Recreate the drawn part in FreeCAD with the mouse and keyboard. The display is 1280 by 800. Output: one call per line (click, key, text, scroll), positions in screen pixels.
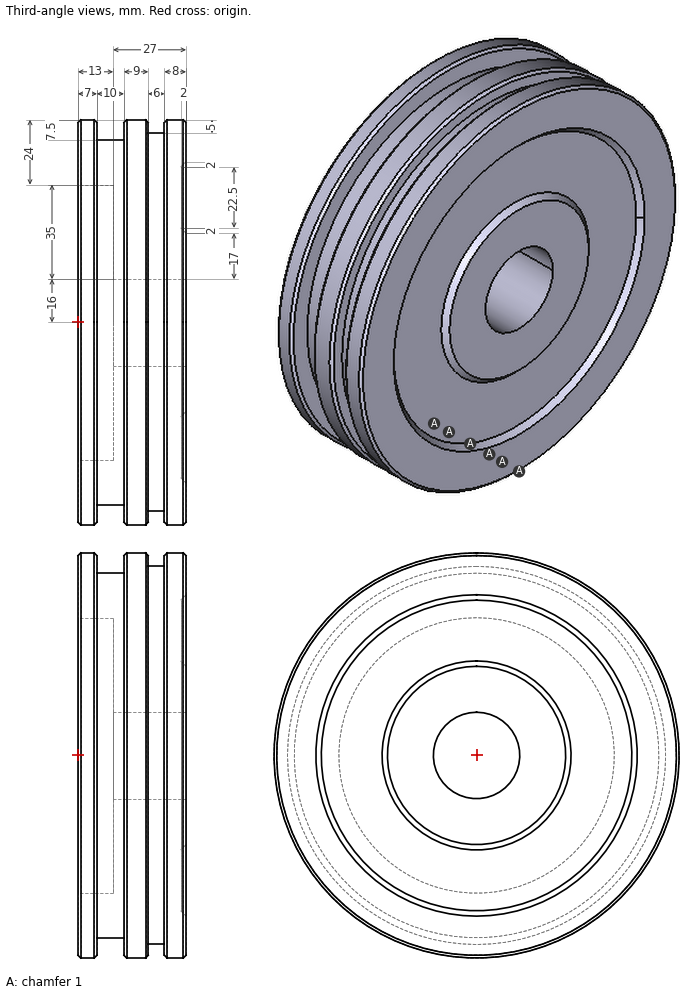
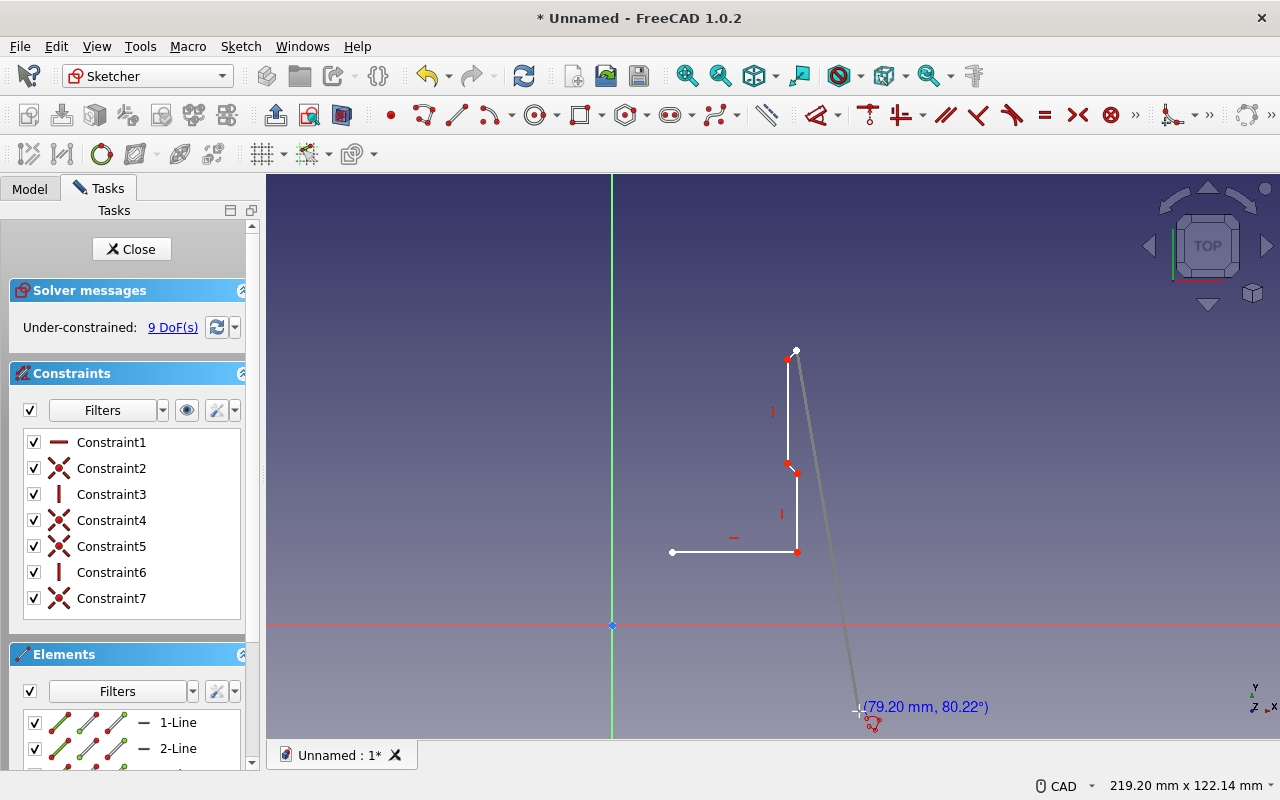
click(797, 278)
click(760, 278)
click(760, 301)
click(732, 301)
click(732, 278)
click(691, 278)
click(691, 313)
click(645, 313)
click(645, 278)
click(612, 278)
click(621, 389)
click(672, 389)
click(672, 552)
key(Escape)
key(Escape)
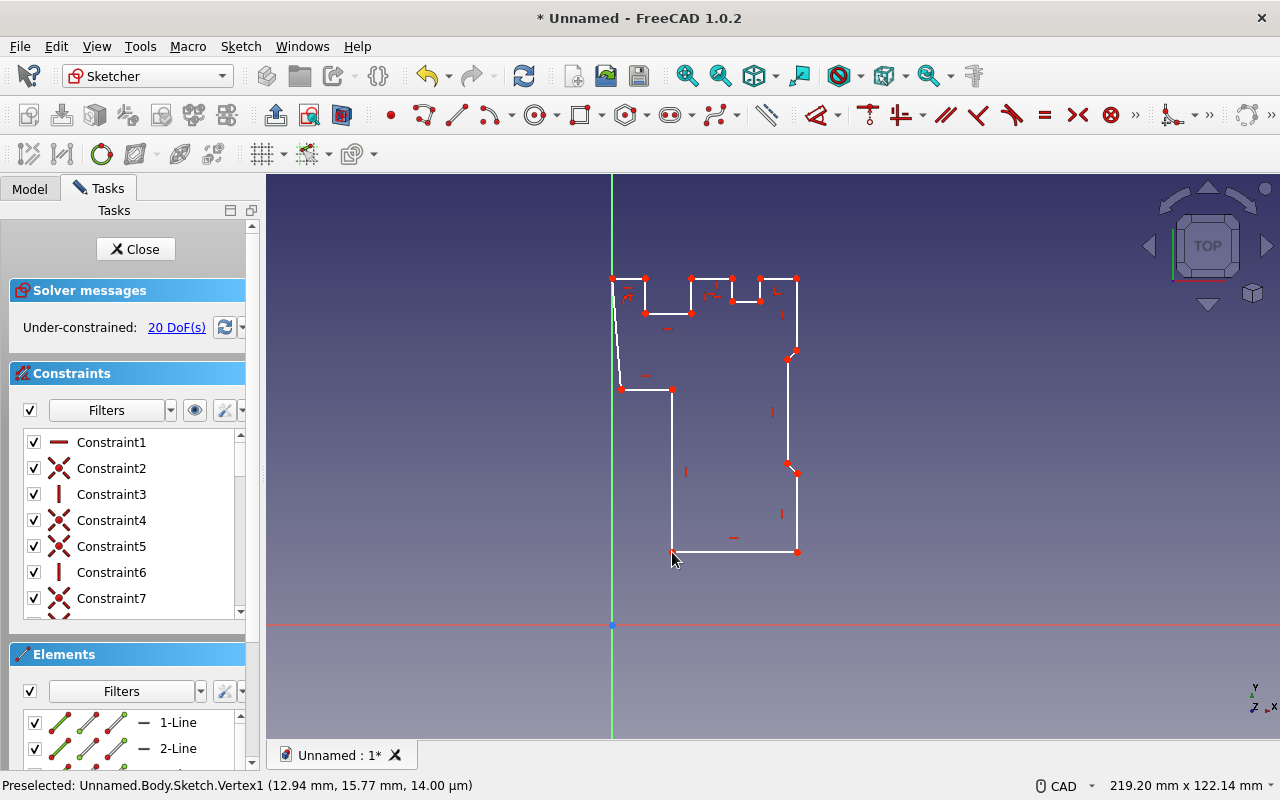
click(615, 312)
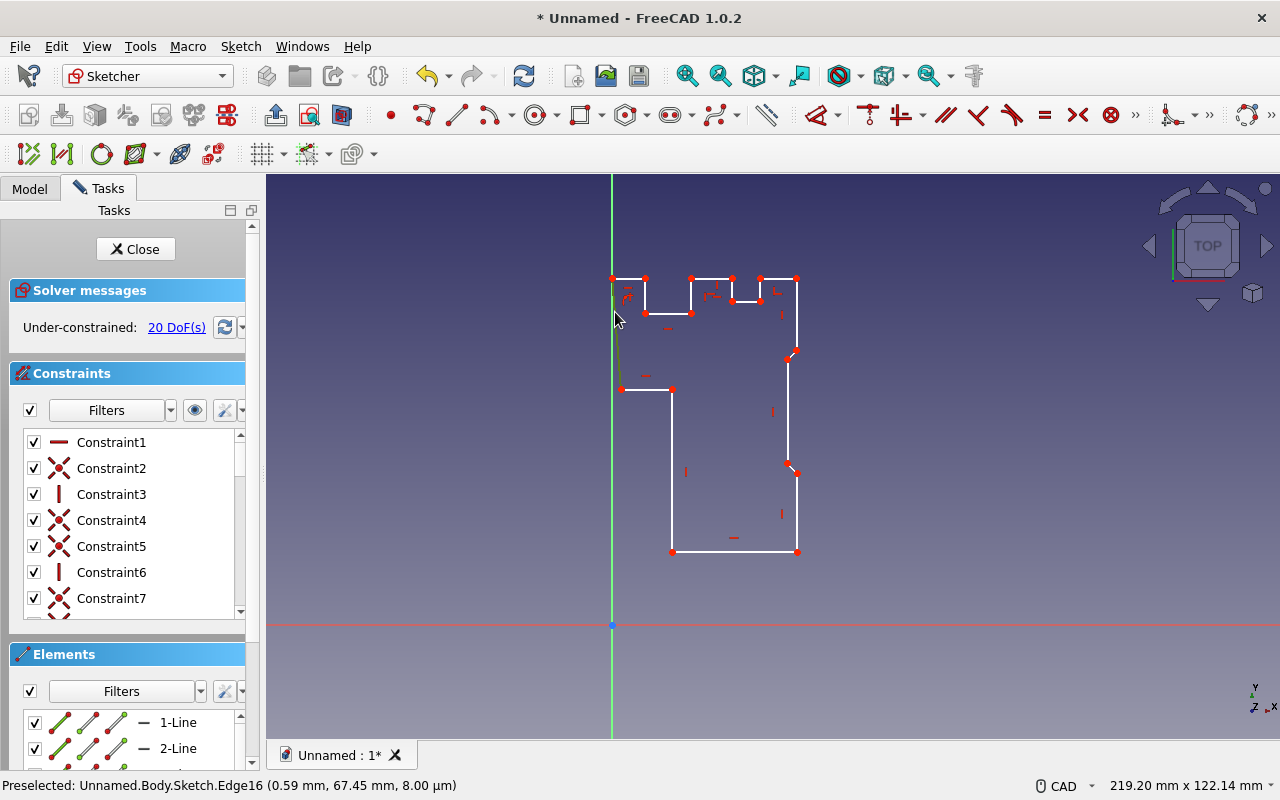
click(922, 116)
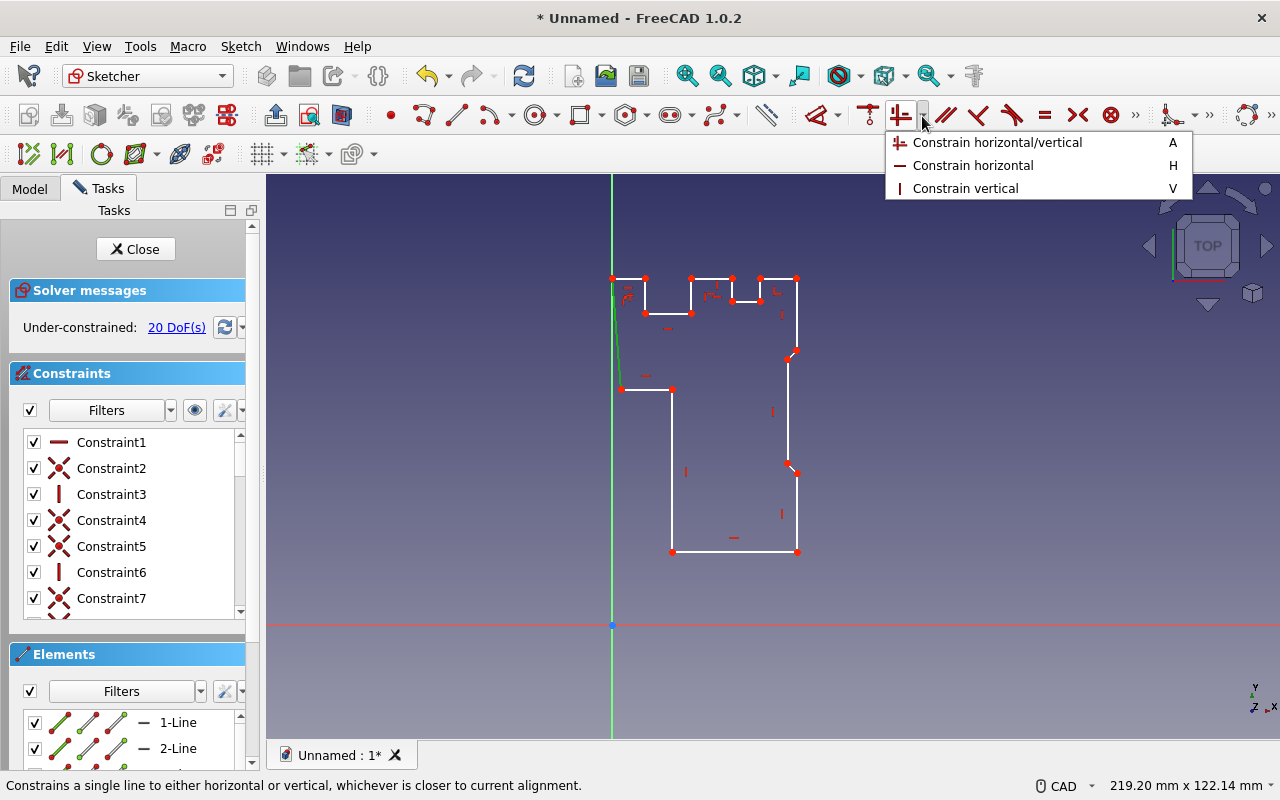
click(1039, 188)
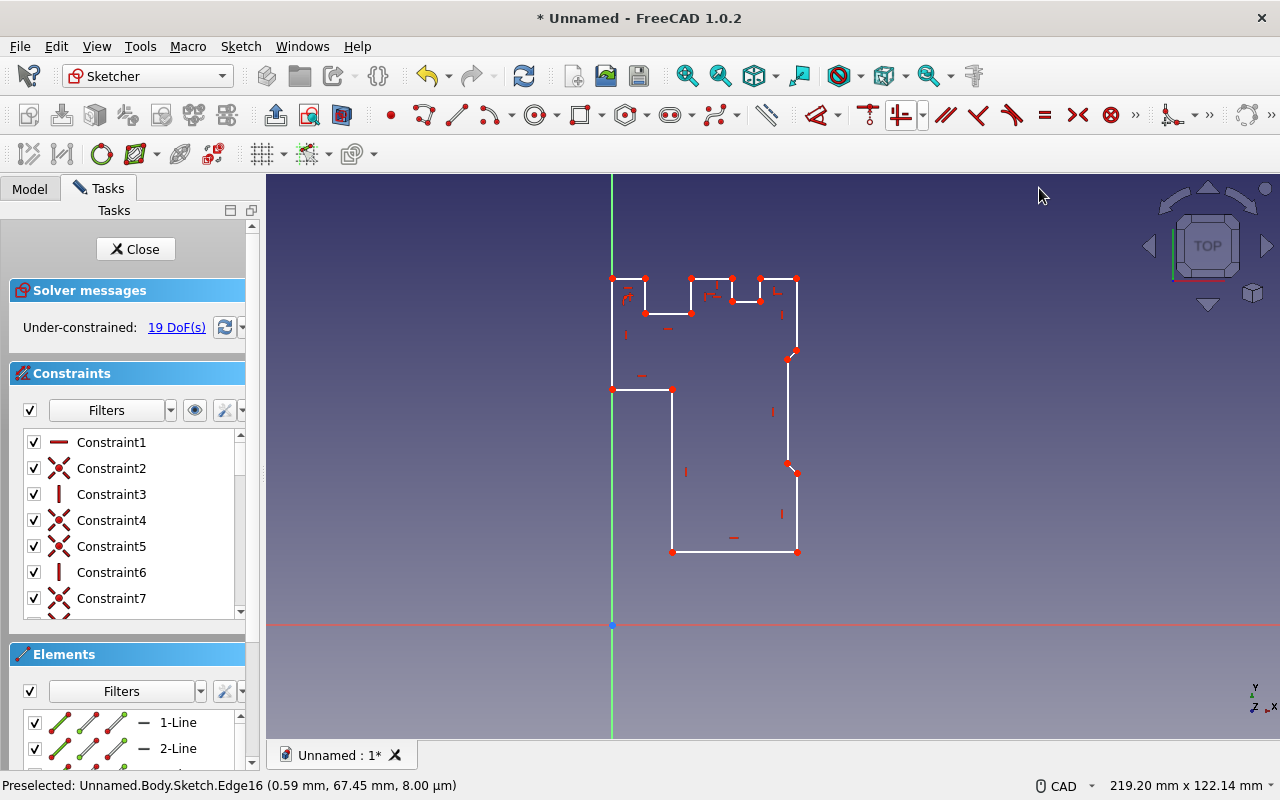
click(816, 116)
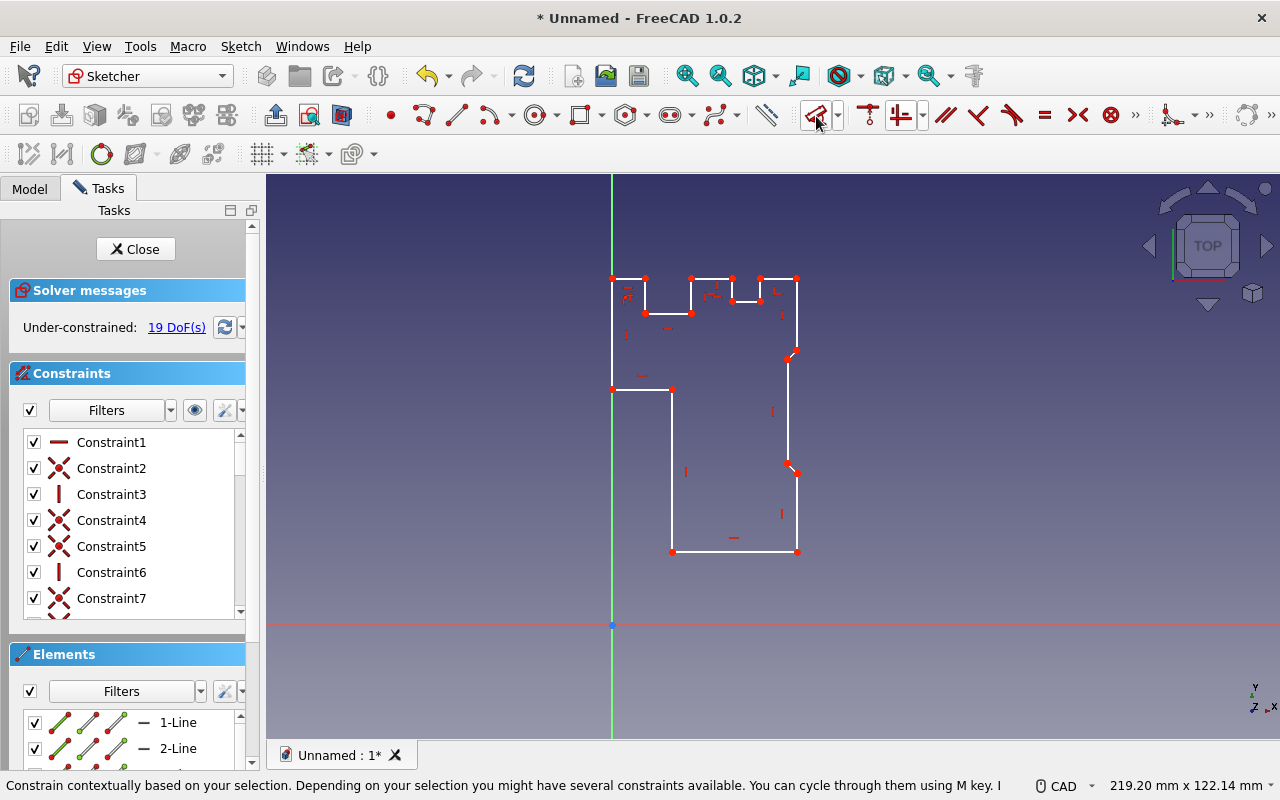
scroll(786, 279, up, 2)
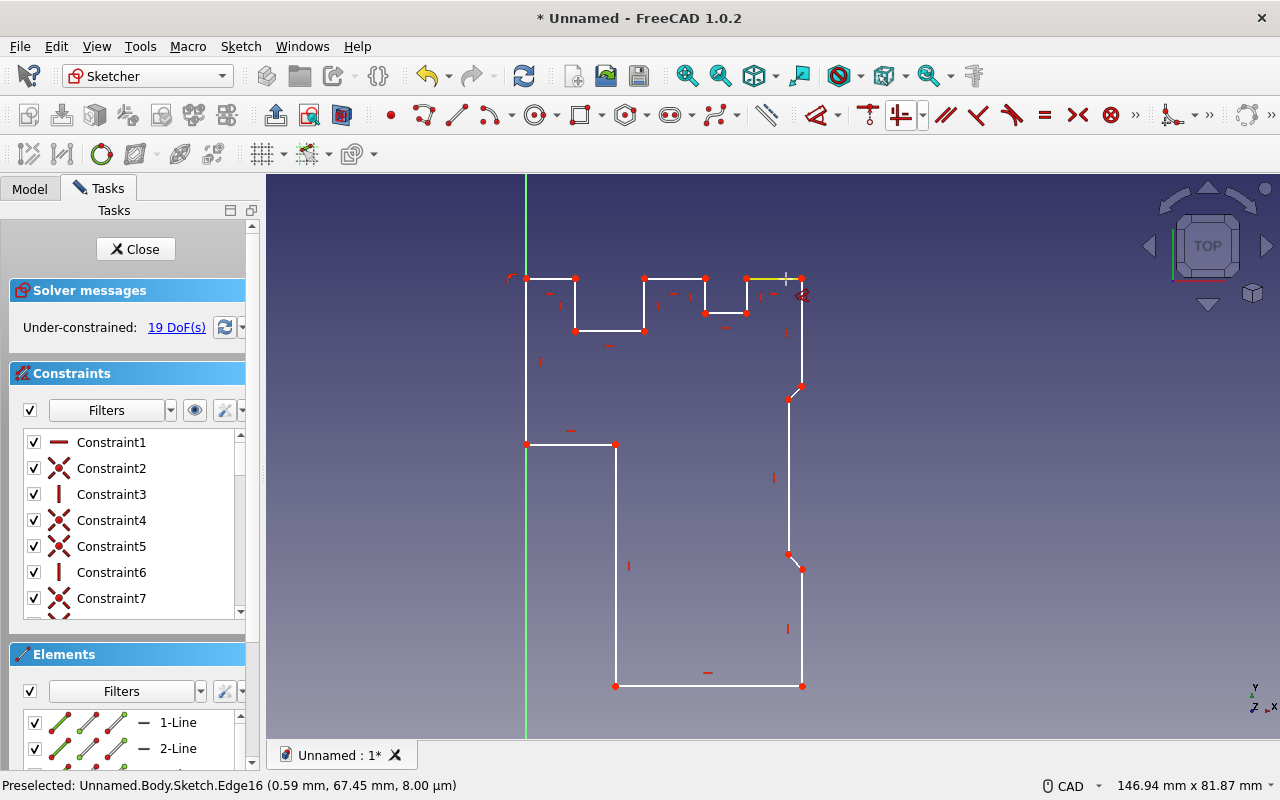
click(785, 279)
click(774, 245)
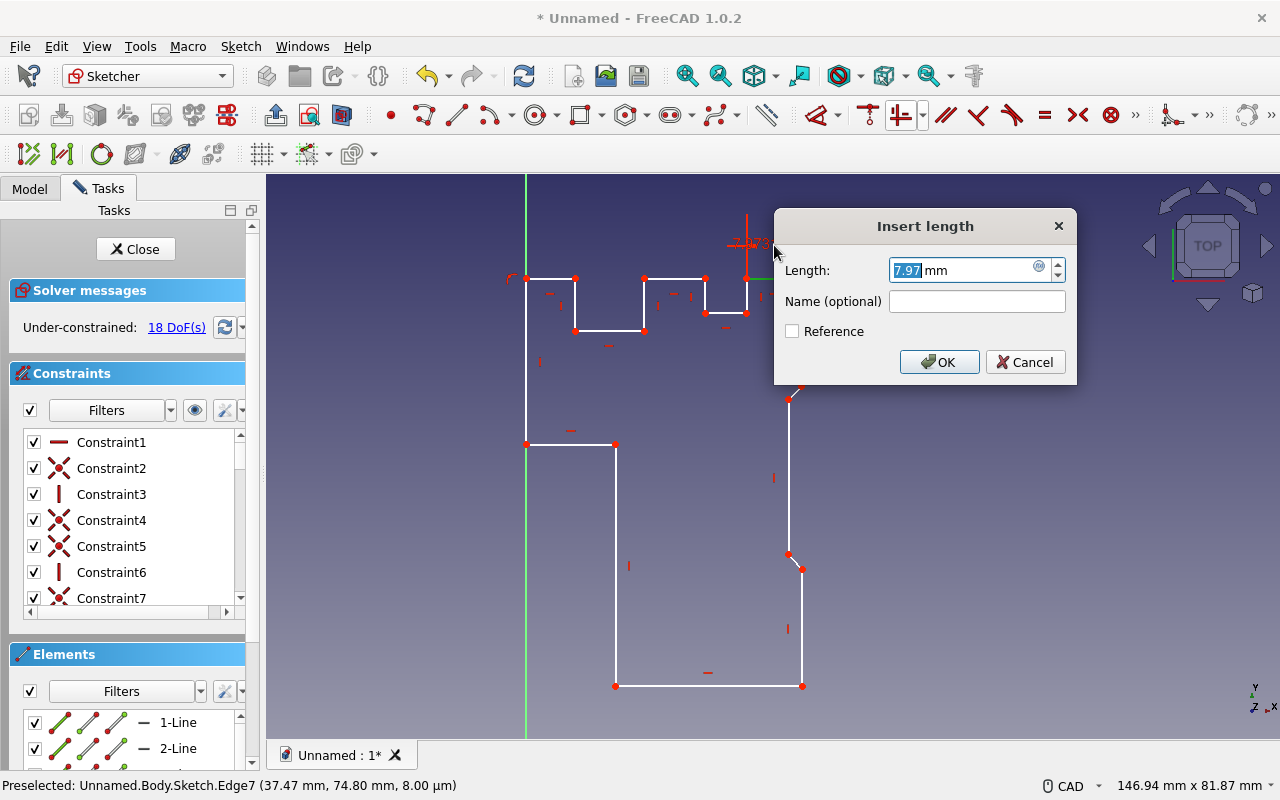
text(8)
key(Return)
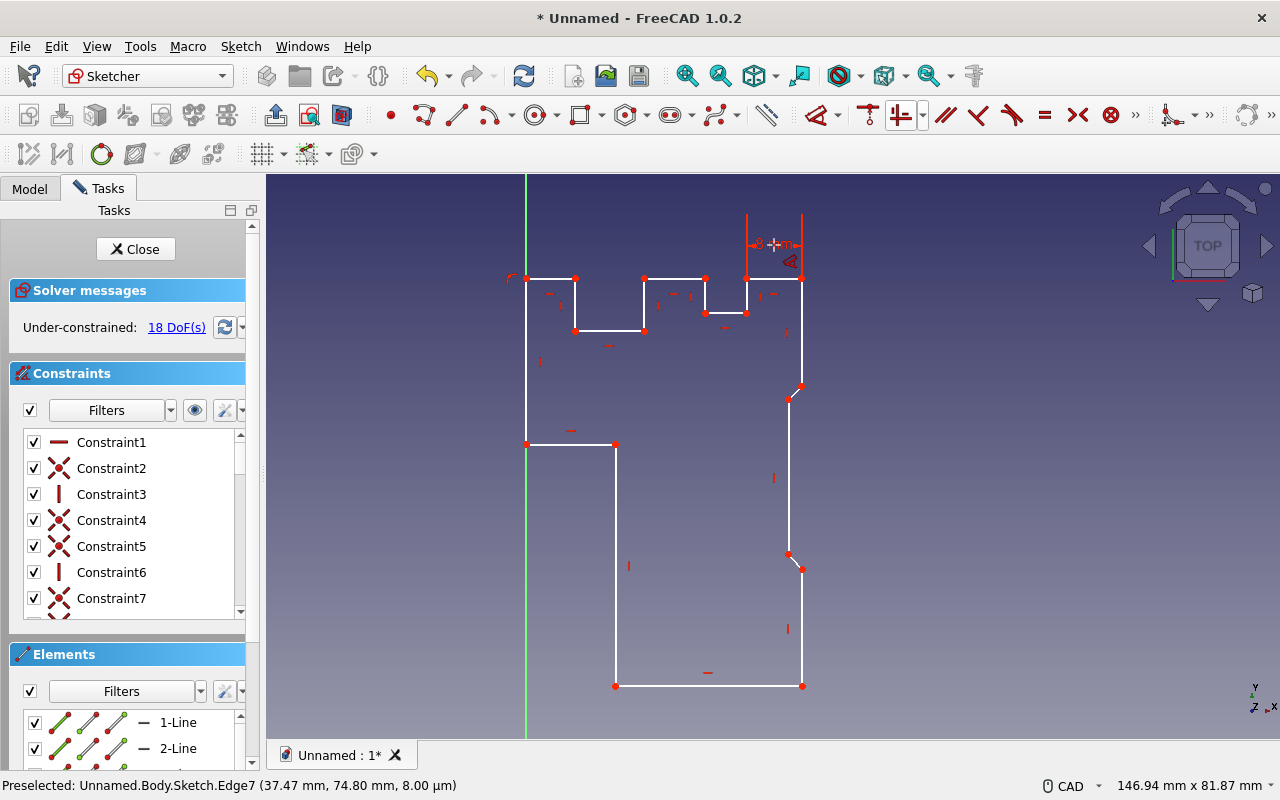
scroll(747, 289, up, 2)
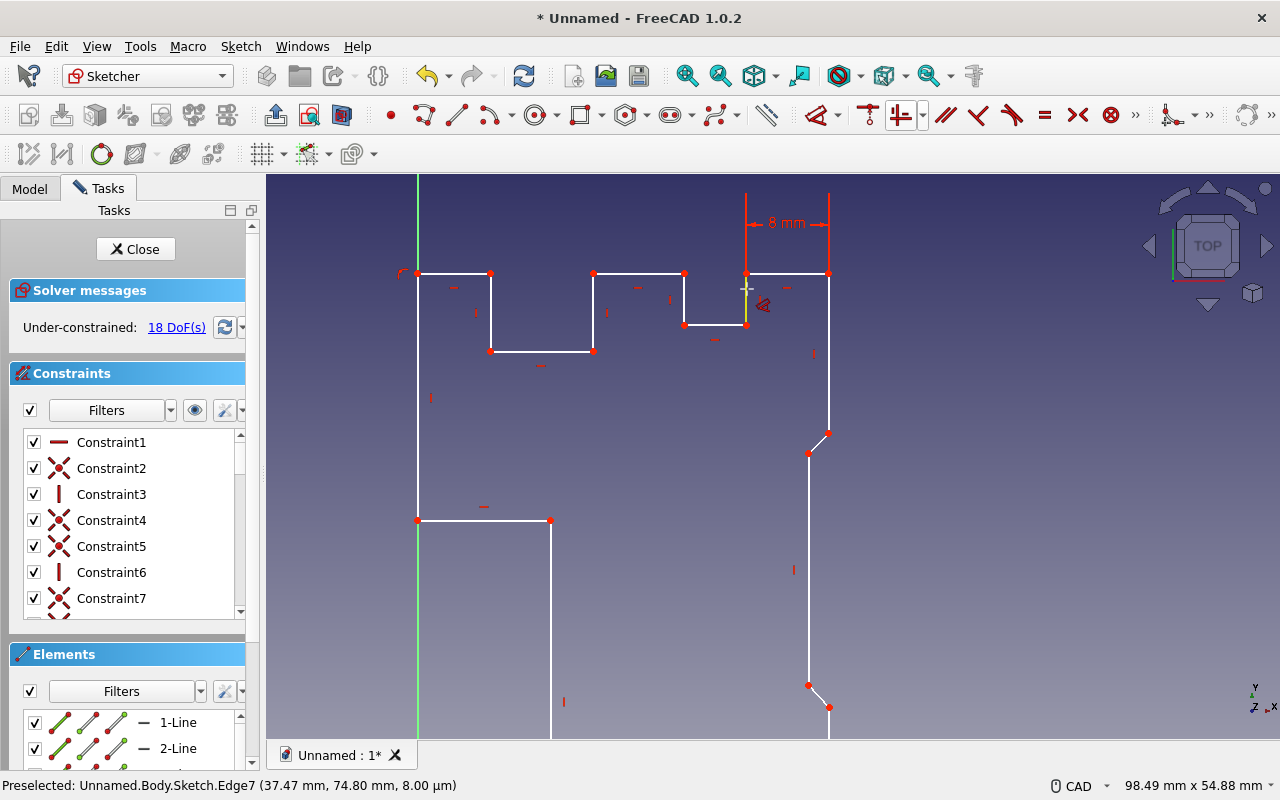
click(746, 289)
click(780, 299)